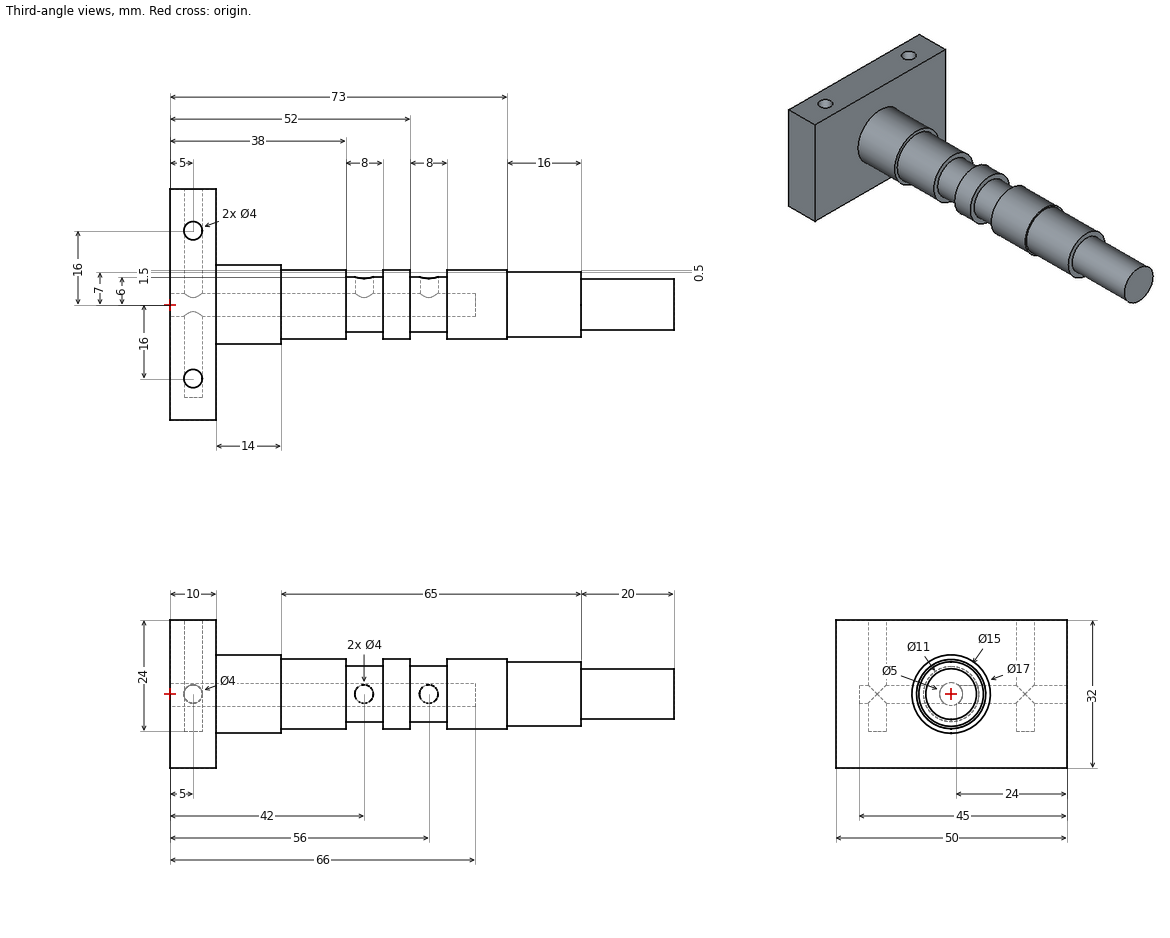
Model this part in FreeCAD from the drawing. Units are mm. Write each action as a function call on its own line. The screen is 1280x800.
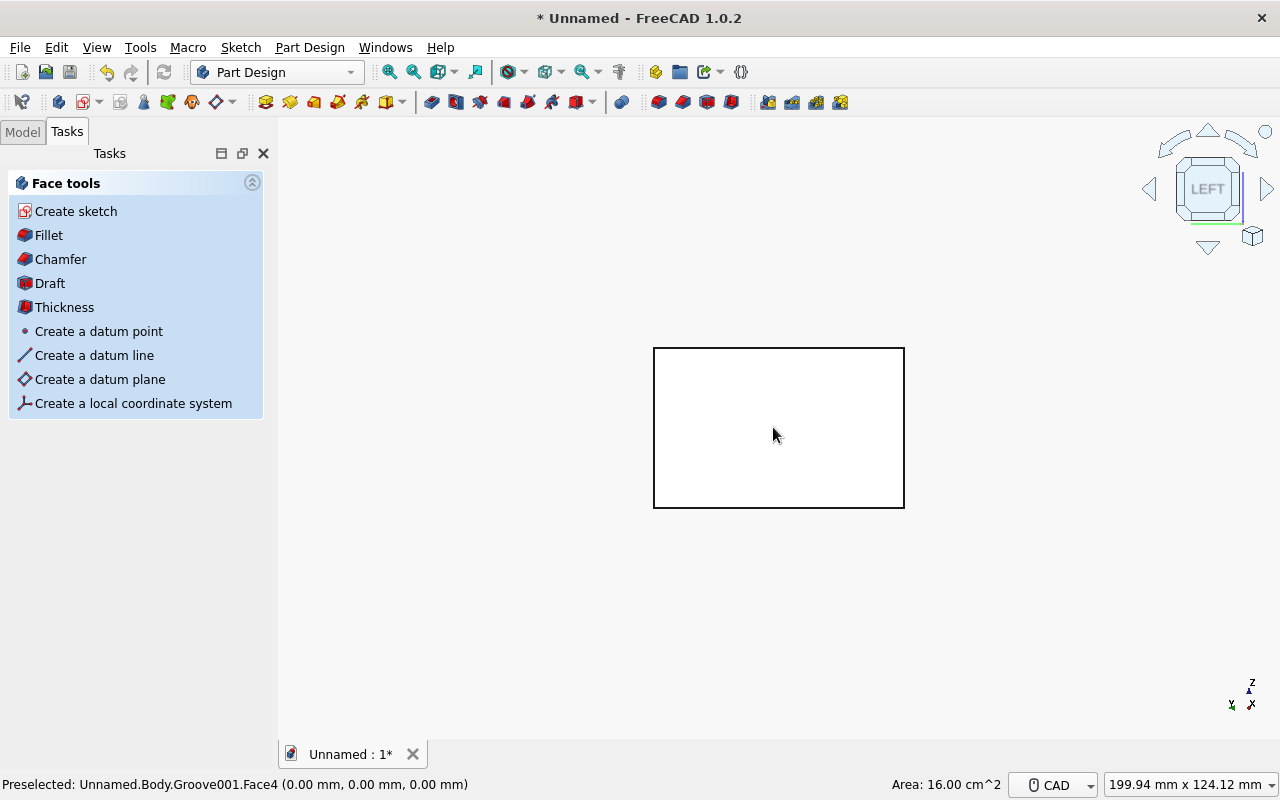
click(84, 102)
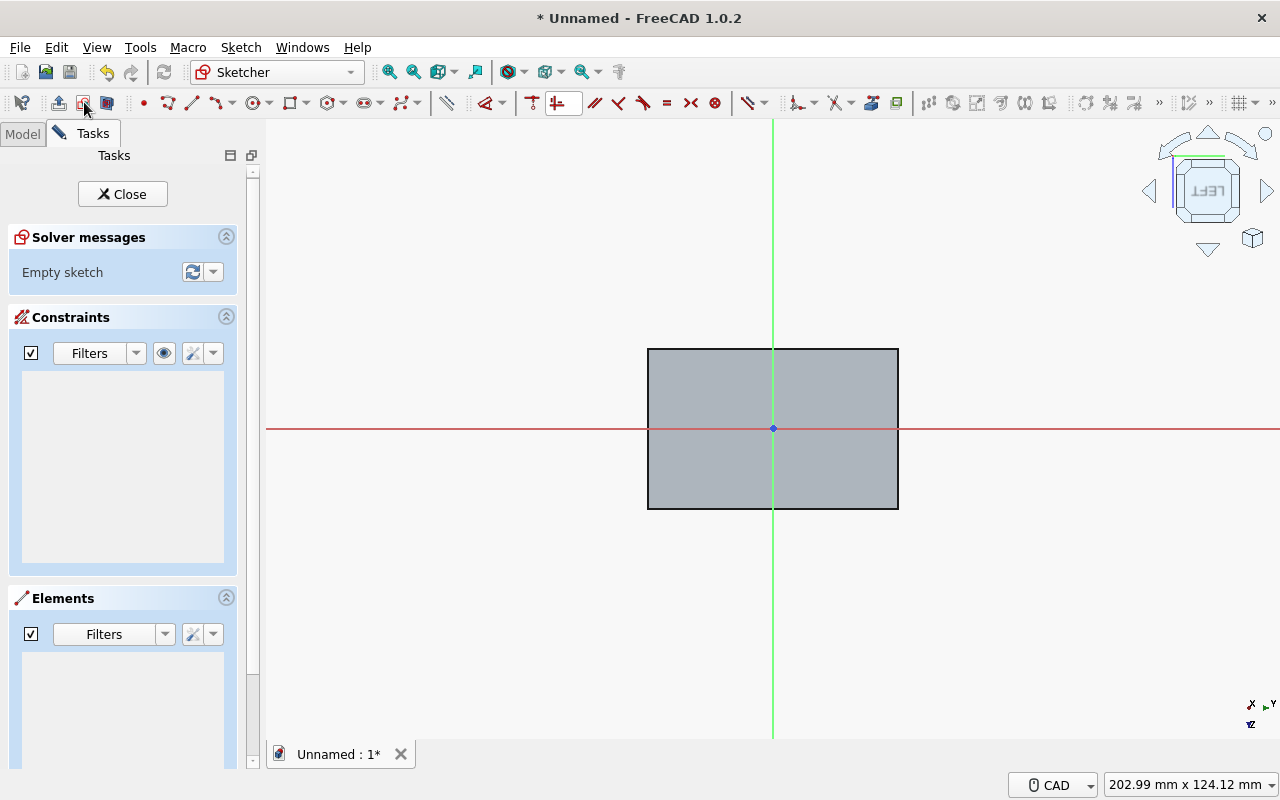
scroll(777, 429, up, 14)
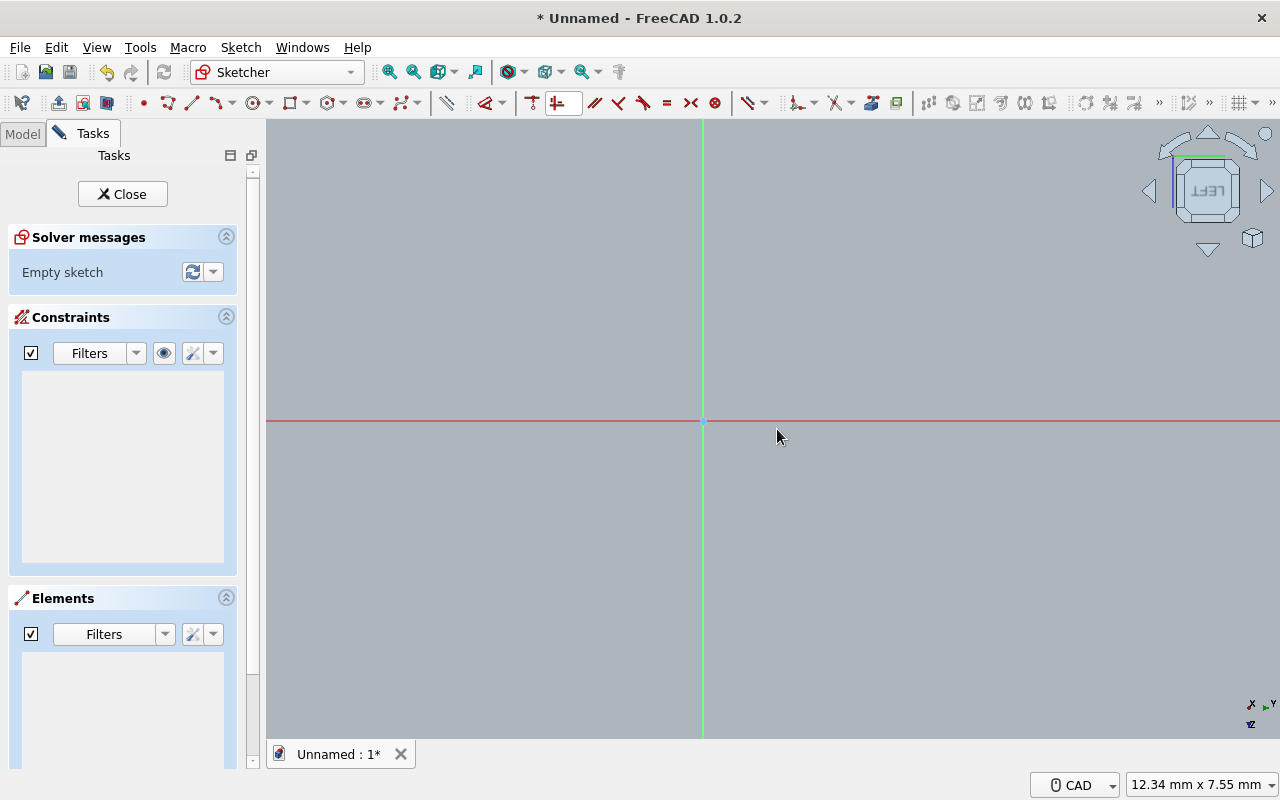
click(254, 104)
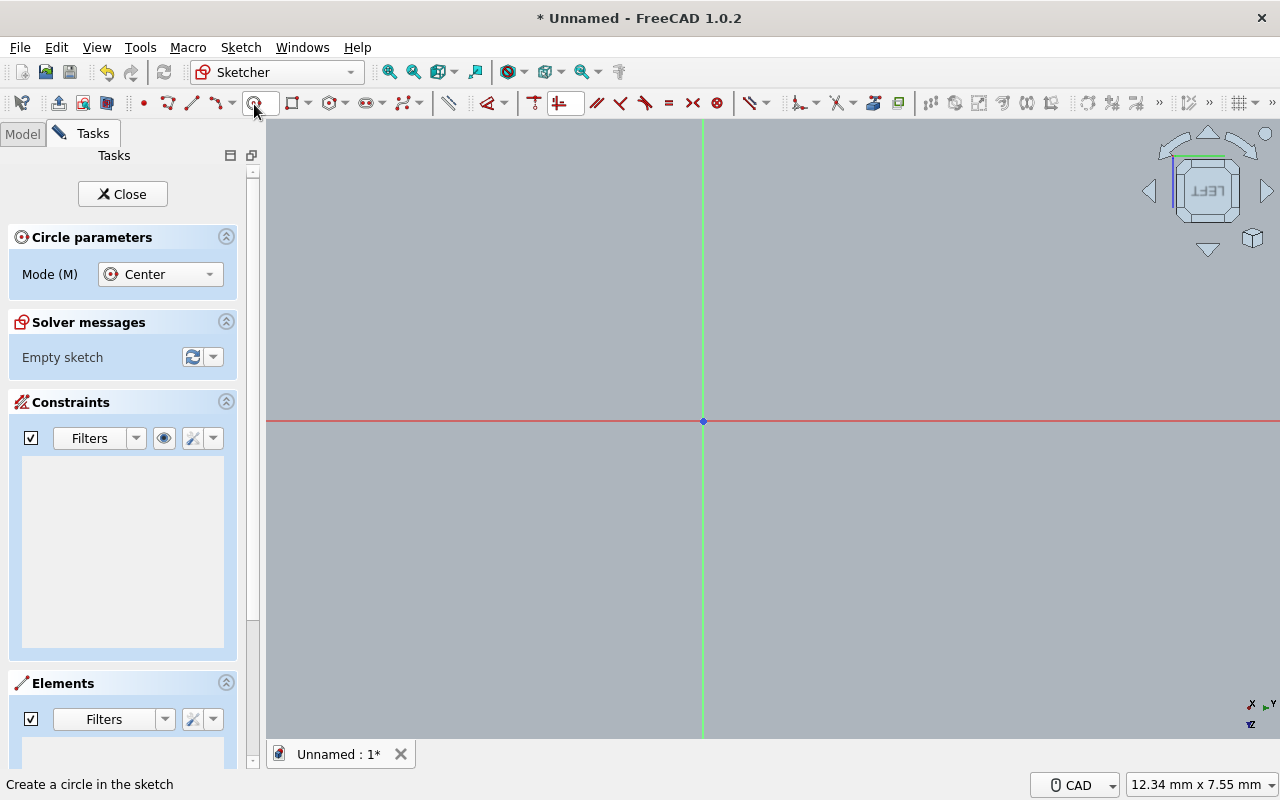
click(703, 421)
move(849, 276)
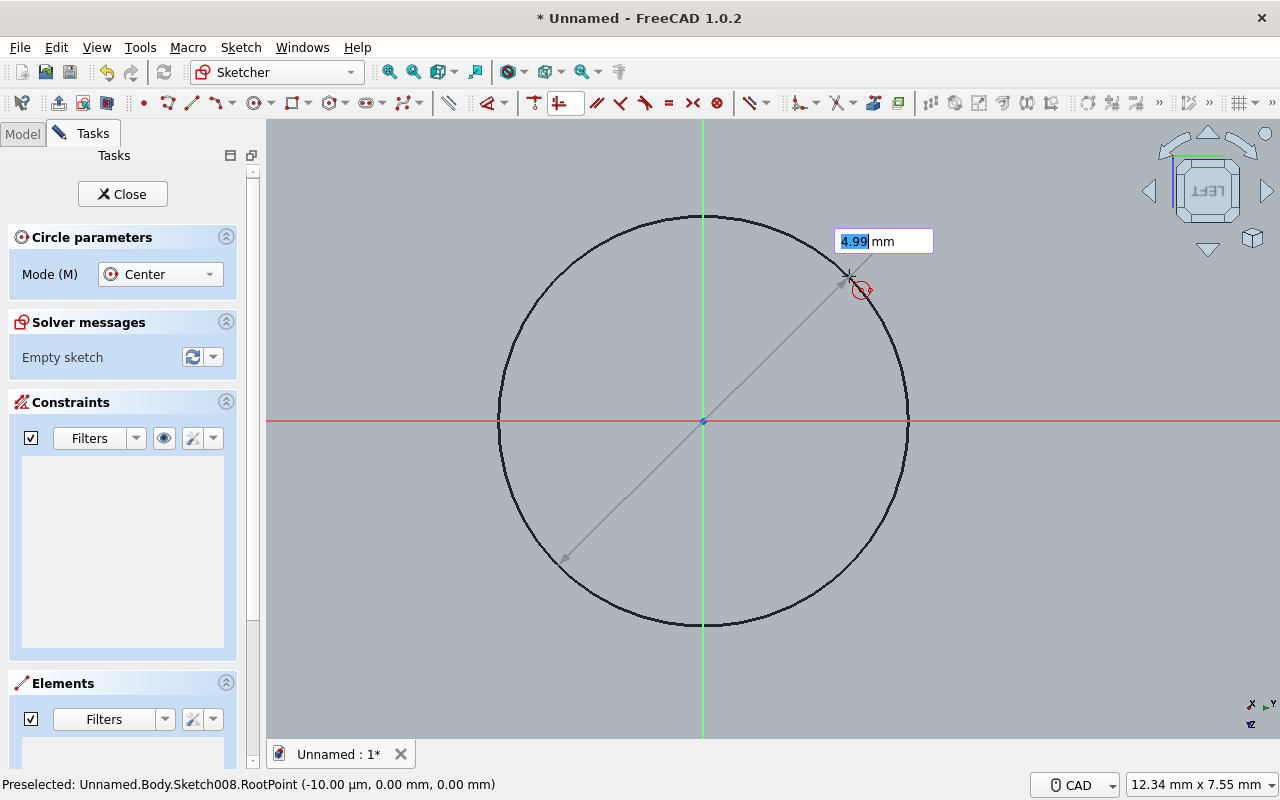
text(5)
key(Return)
key(Escape)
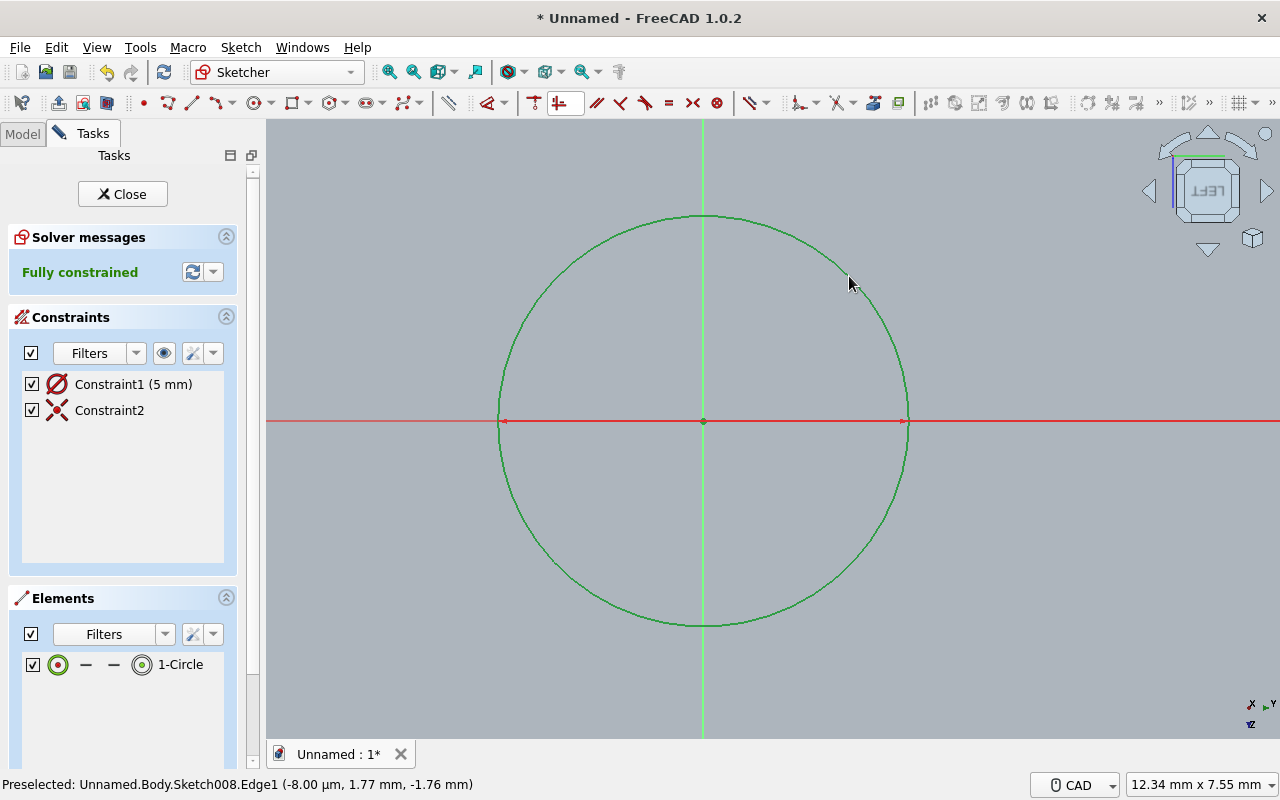
click(123, 194)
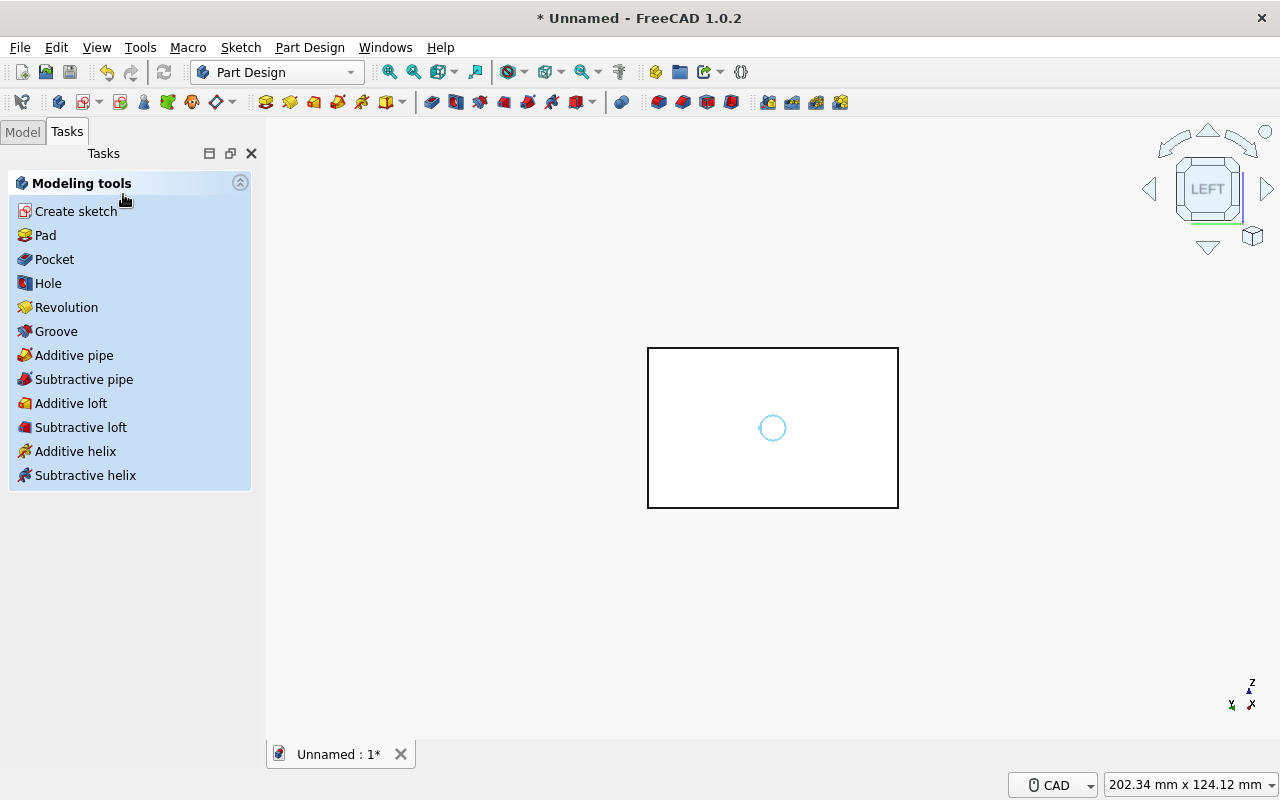
click(432, 102)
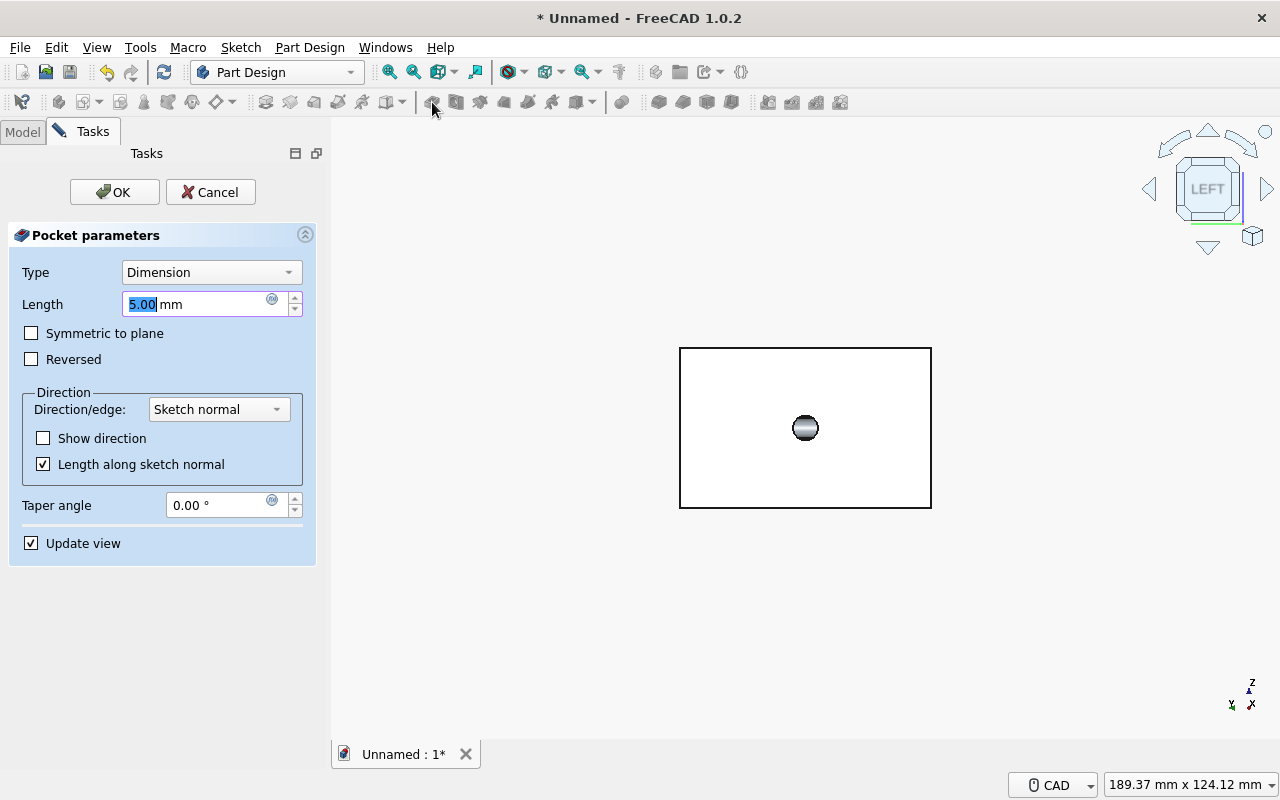
text(66)
key(Tab)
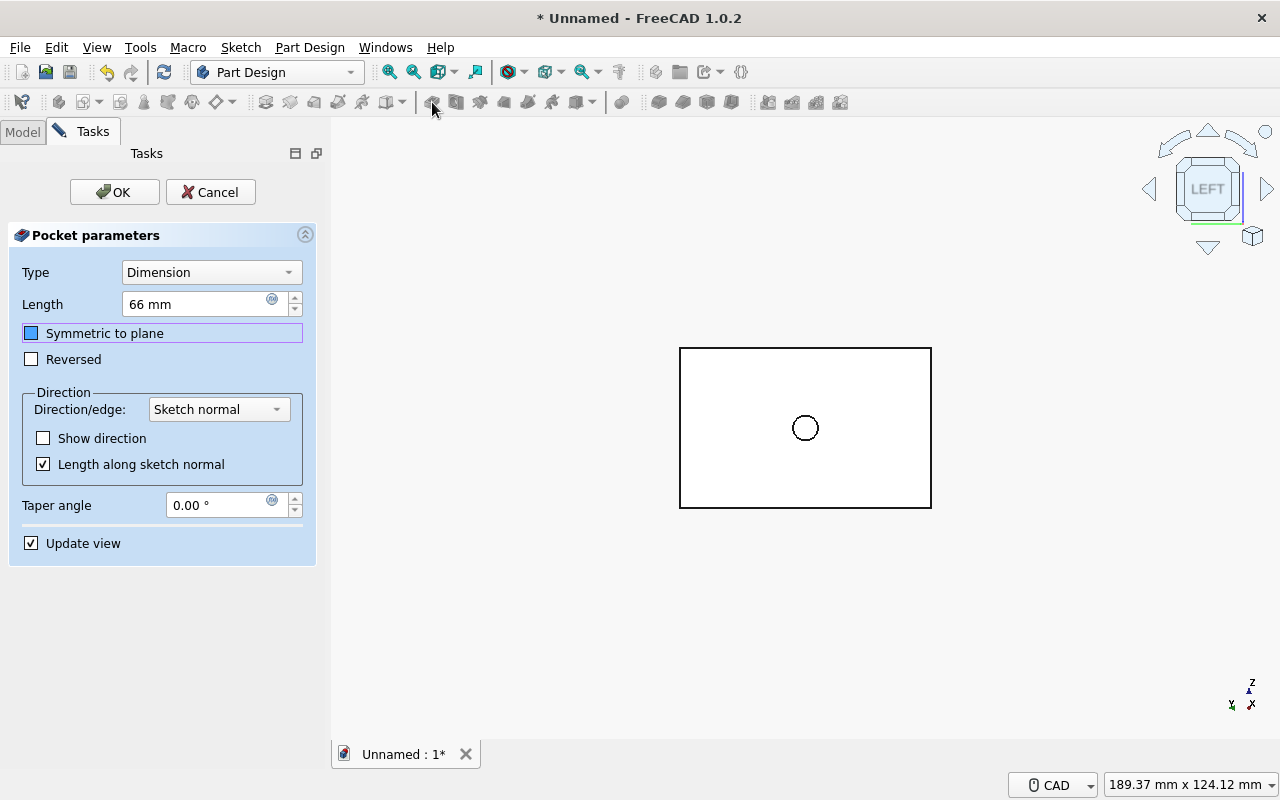
click(115, 192)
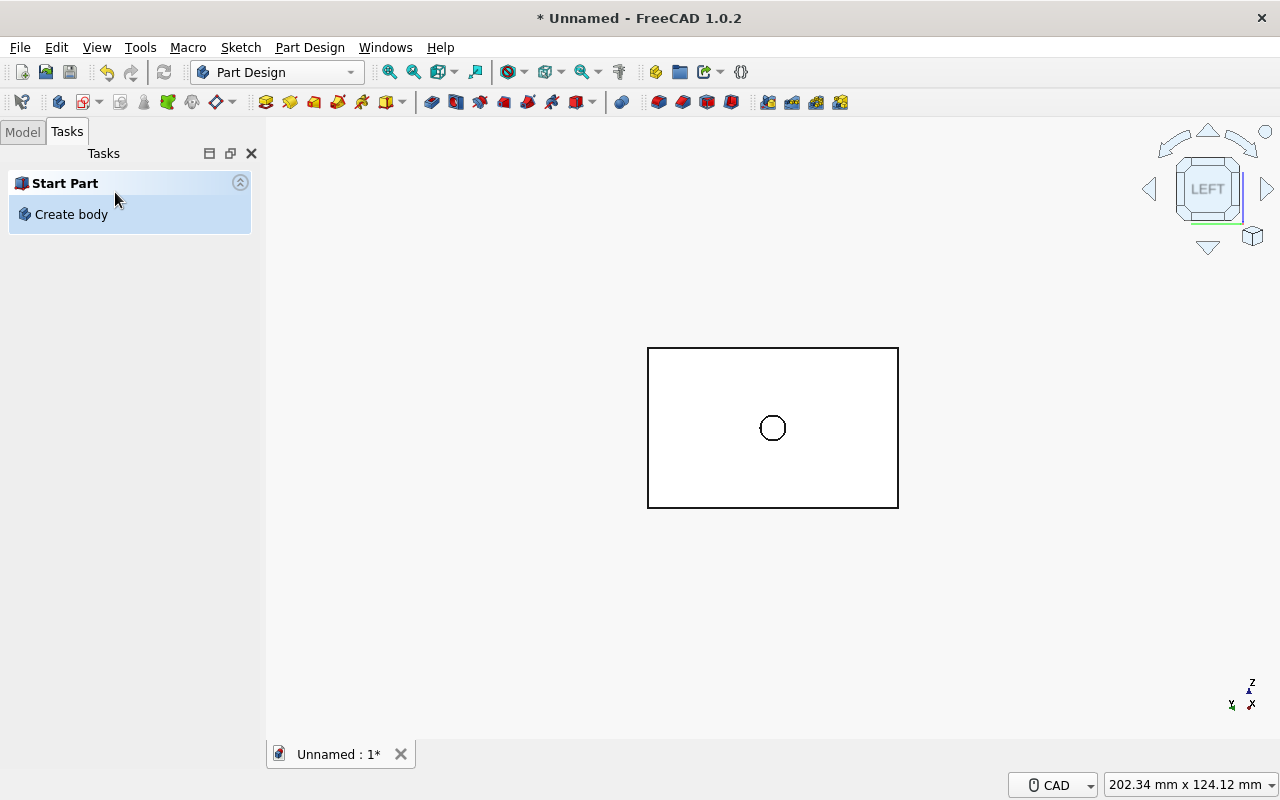
click(390, 72)